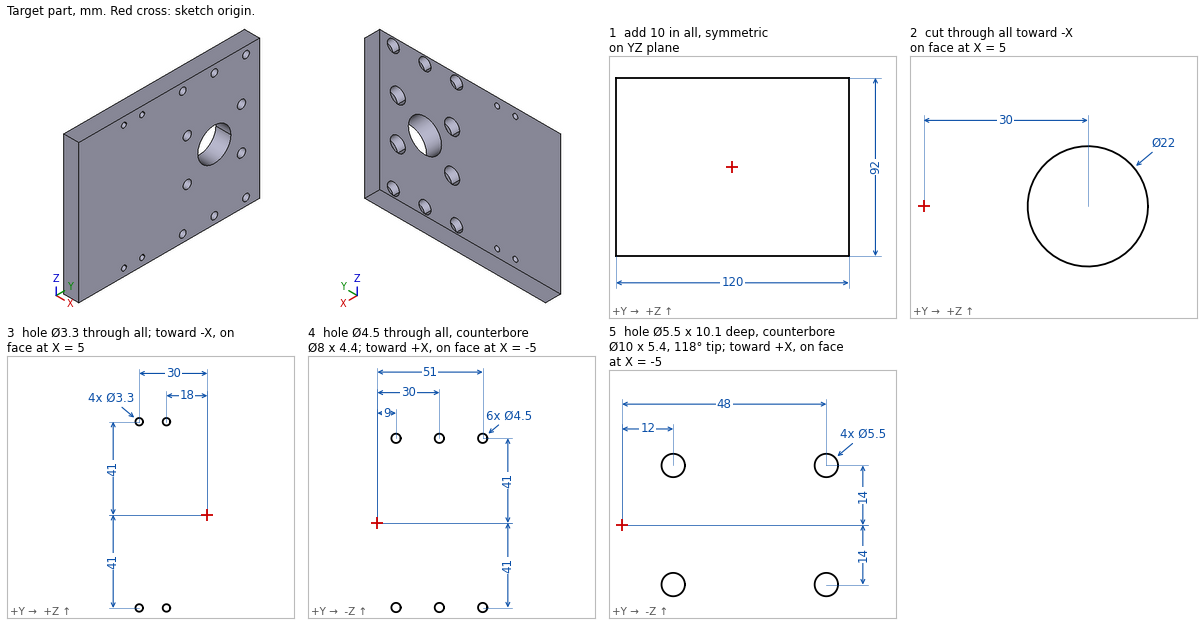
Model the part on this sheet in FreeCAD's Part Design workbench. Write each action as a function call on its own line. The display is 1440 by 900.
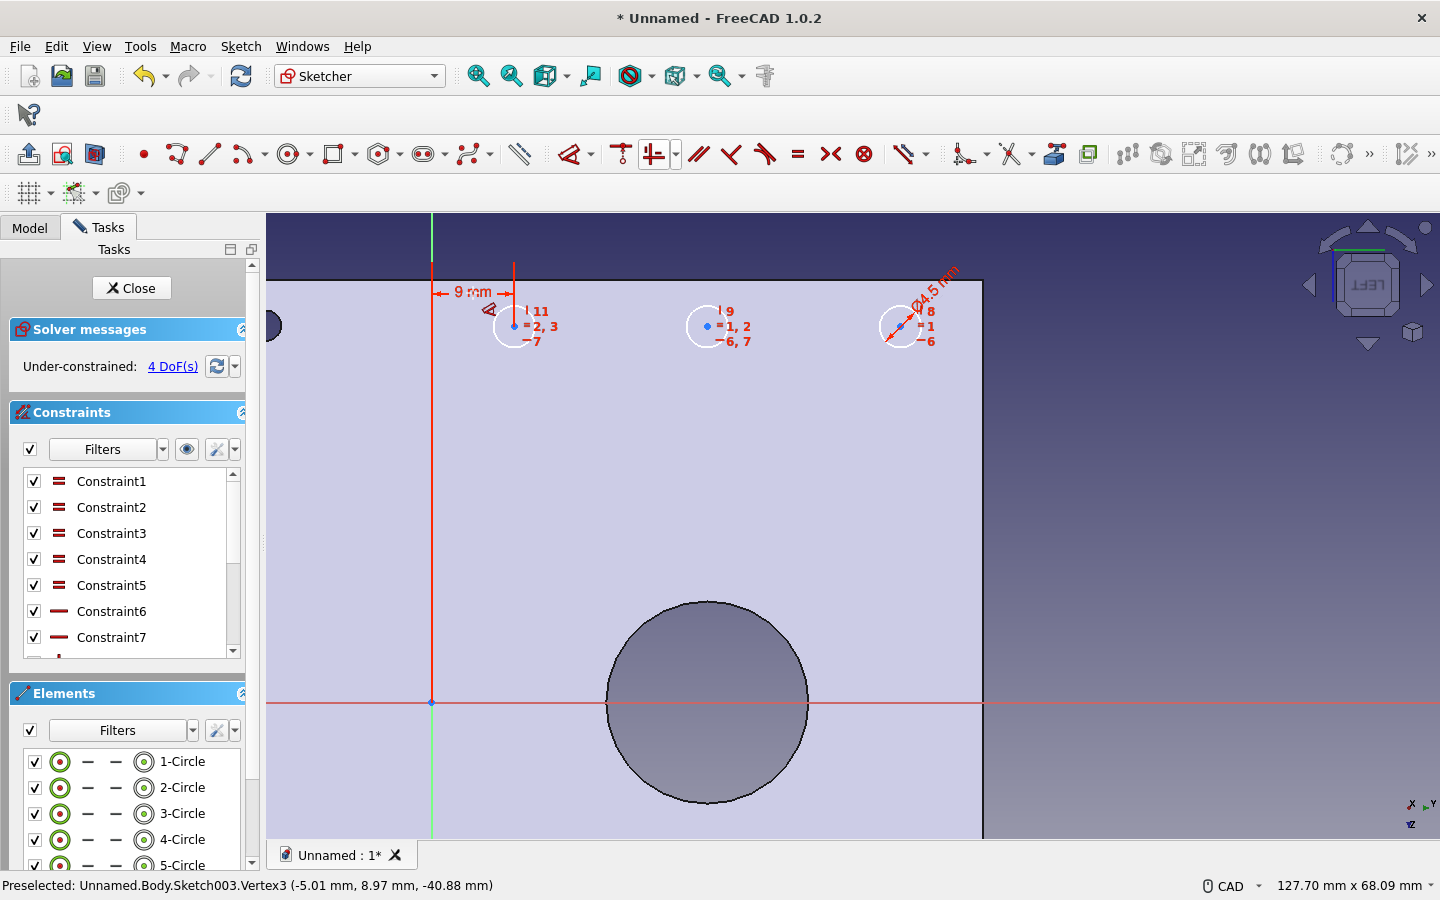
click(900, 327)
click(666, 293)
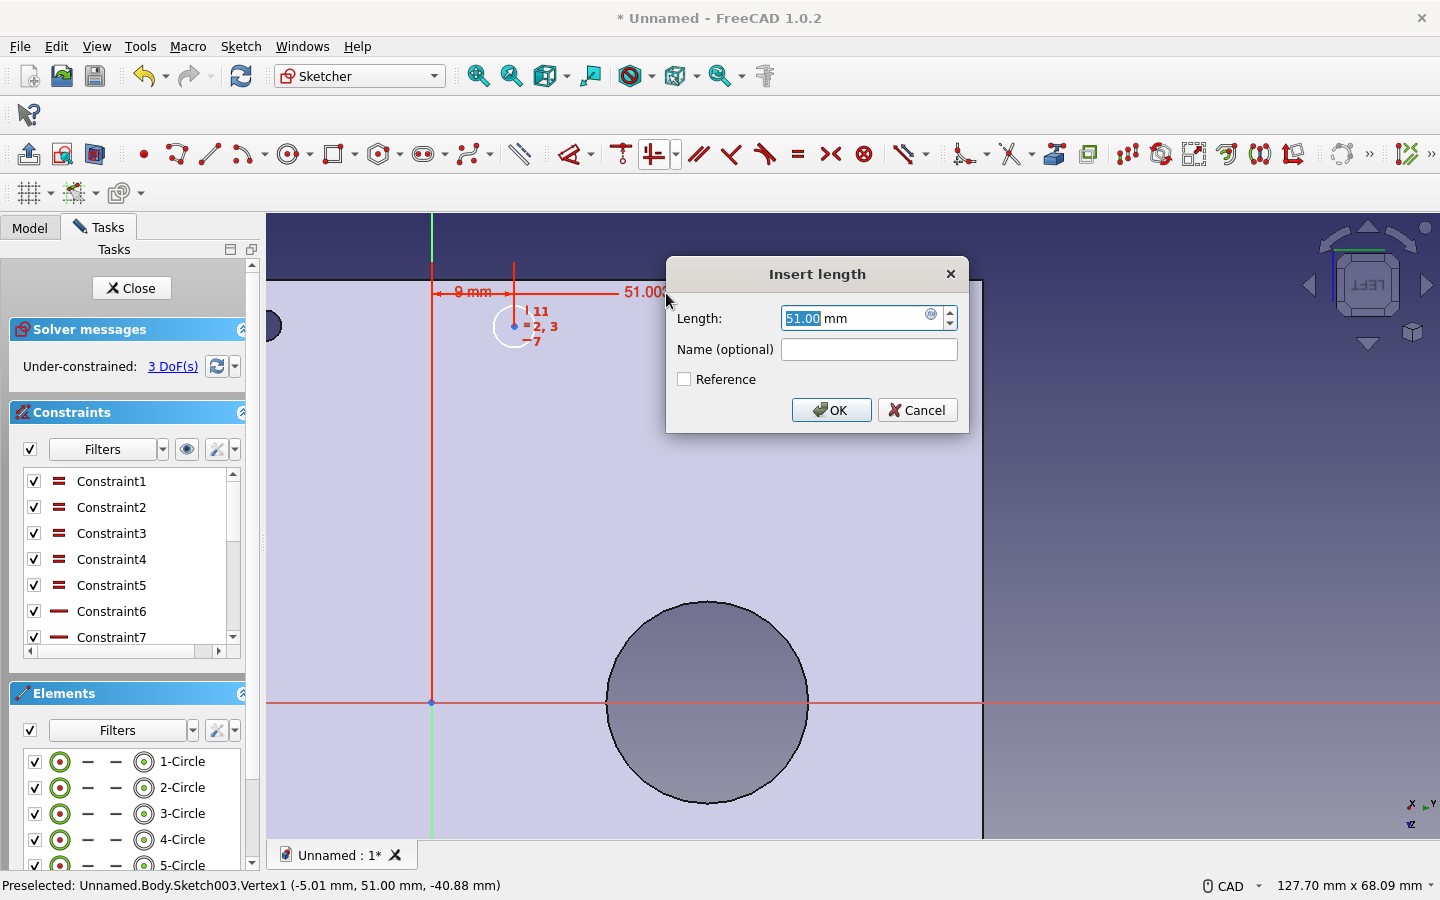
text(51)
key(Return)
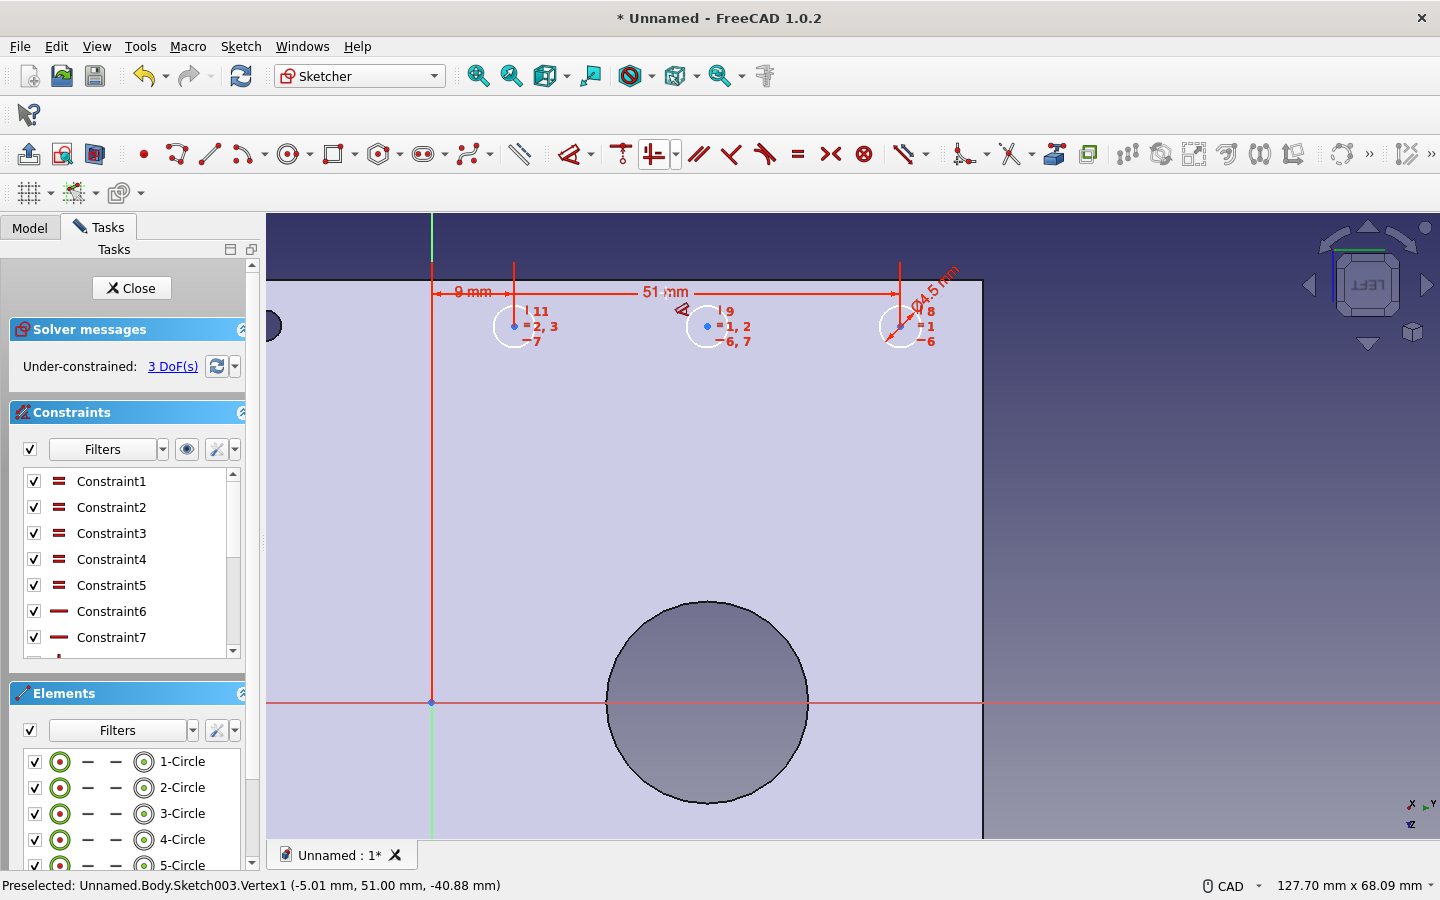
click(900, 327)
click(398, 515)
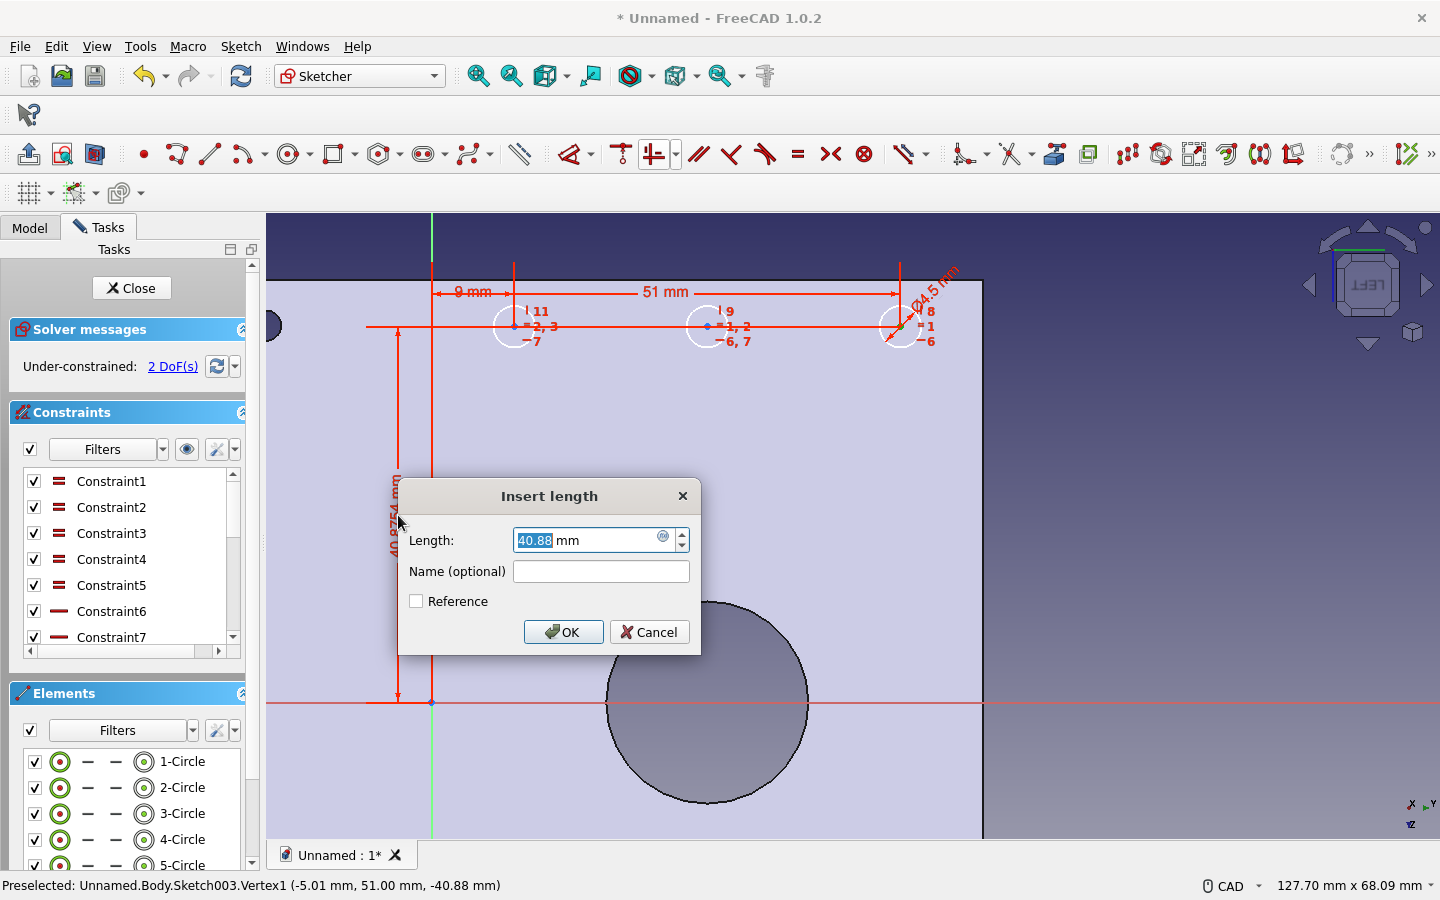
text(41)
key(Return)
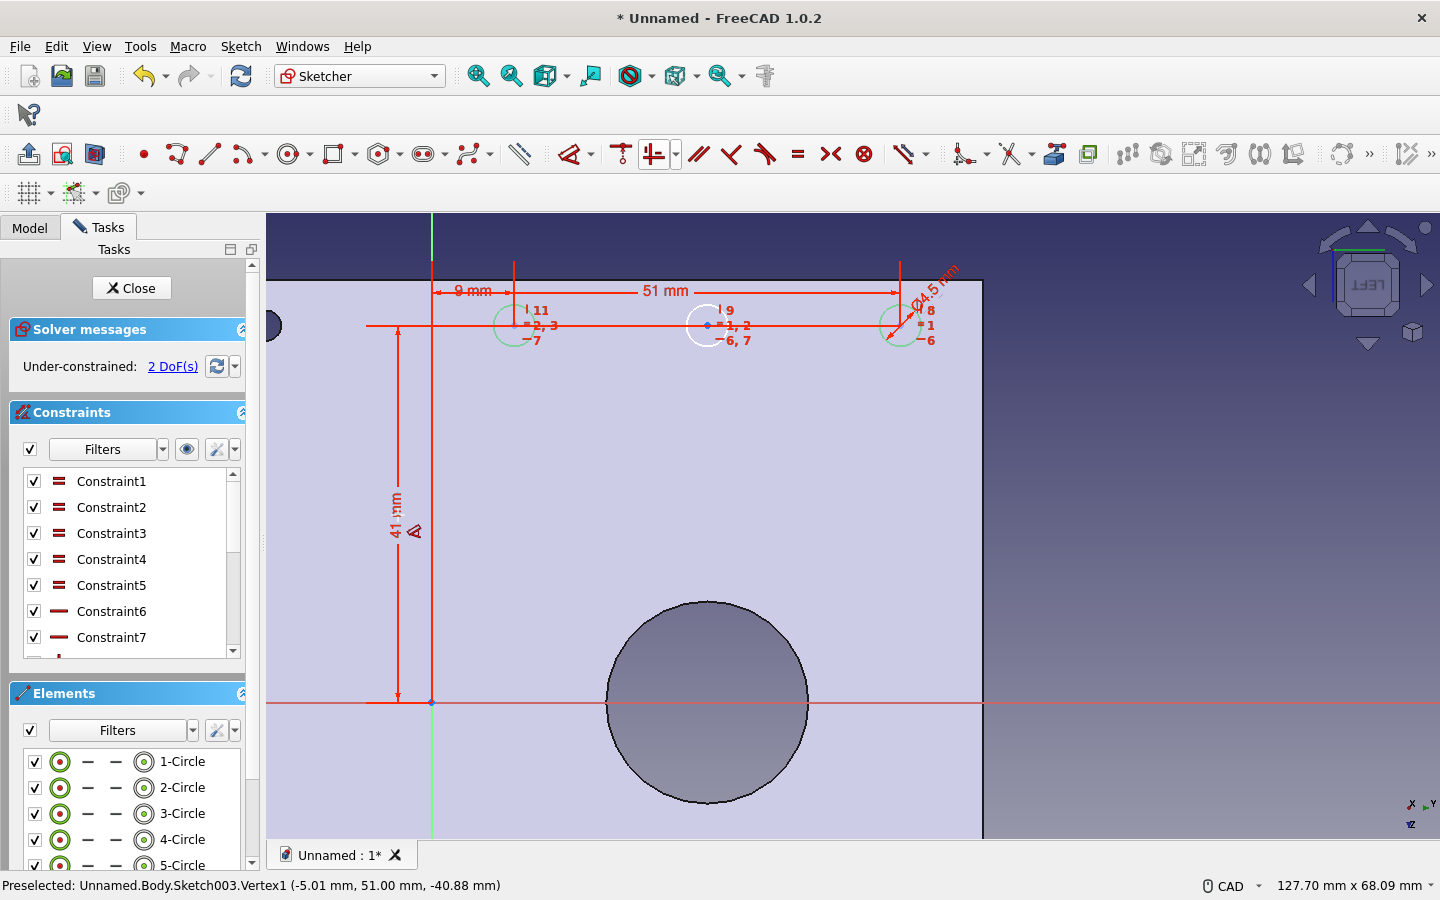
click(707, 326)
click(569, 292)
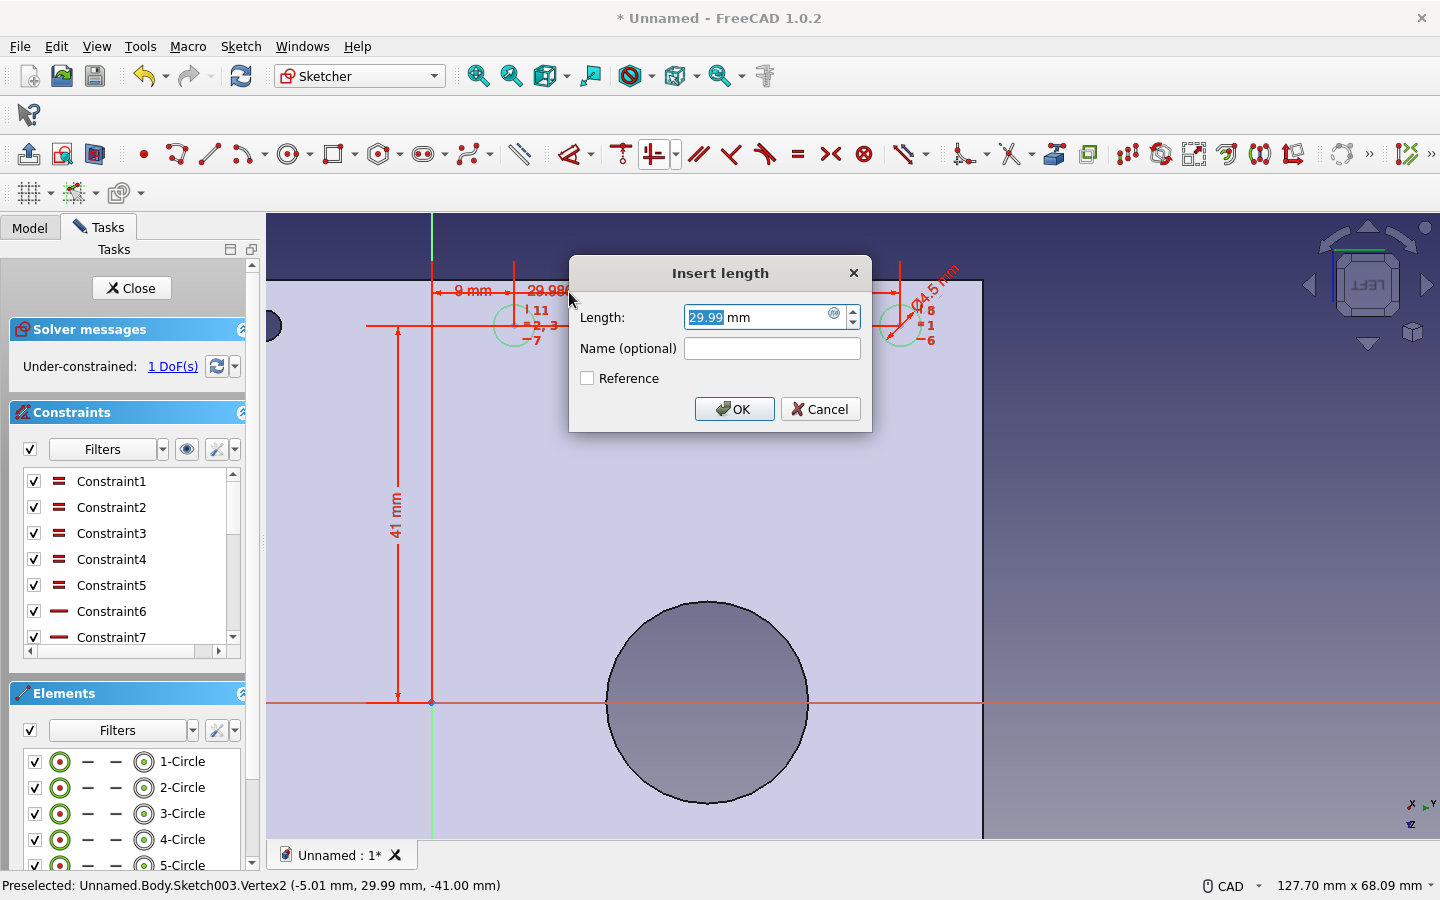
text(30)
key(Return)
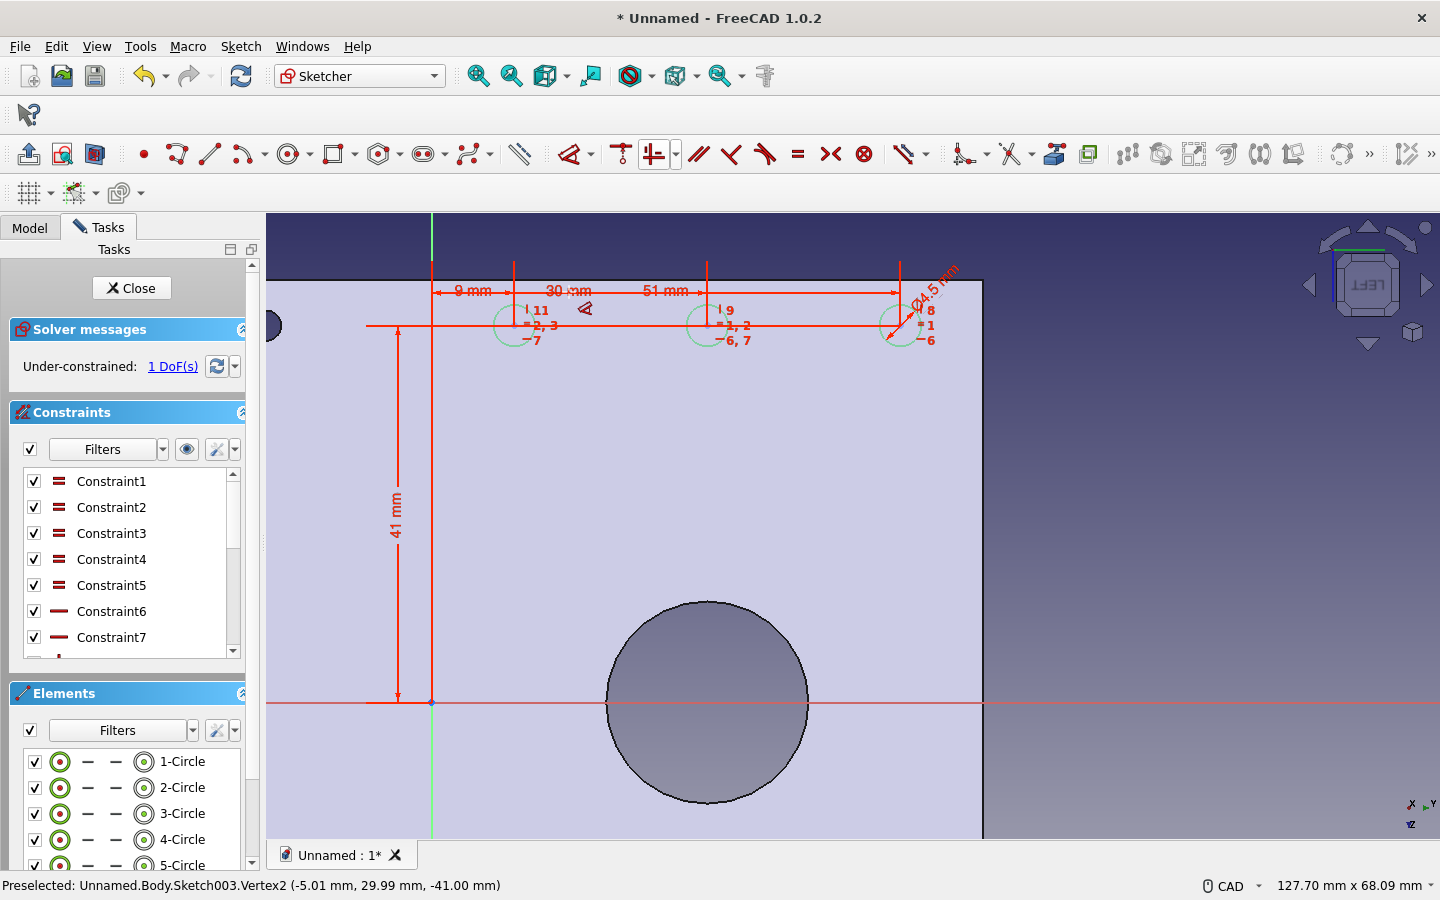
scroll(916, 311, down, 3)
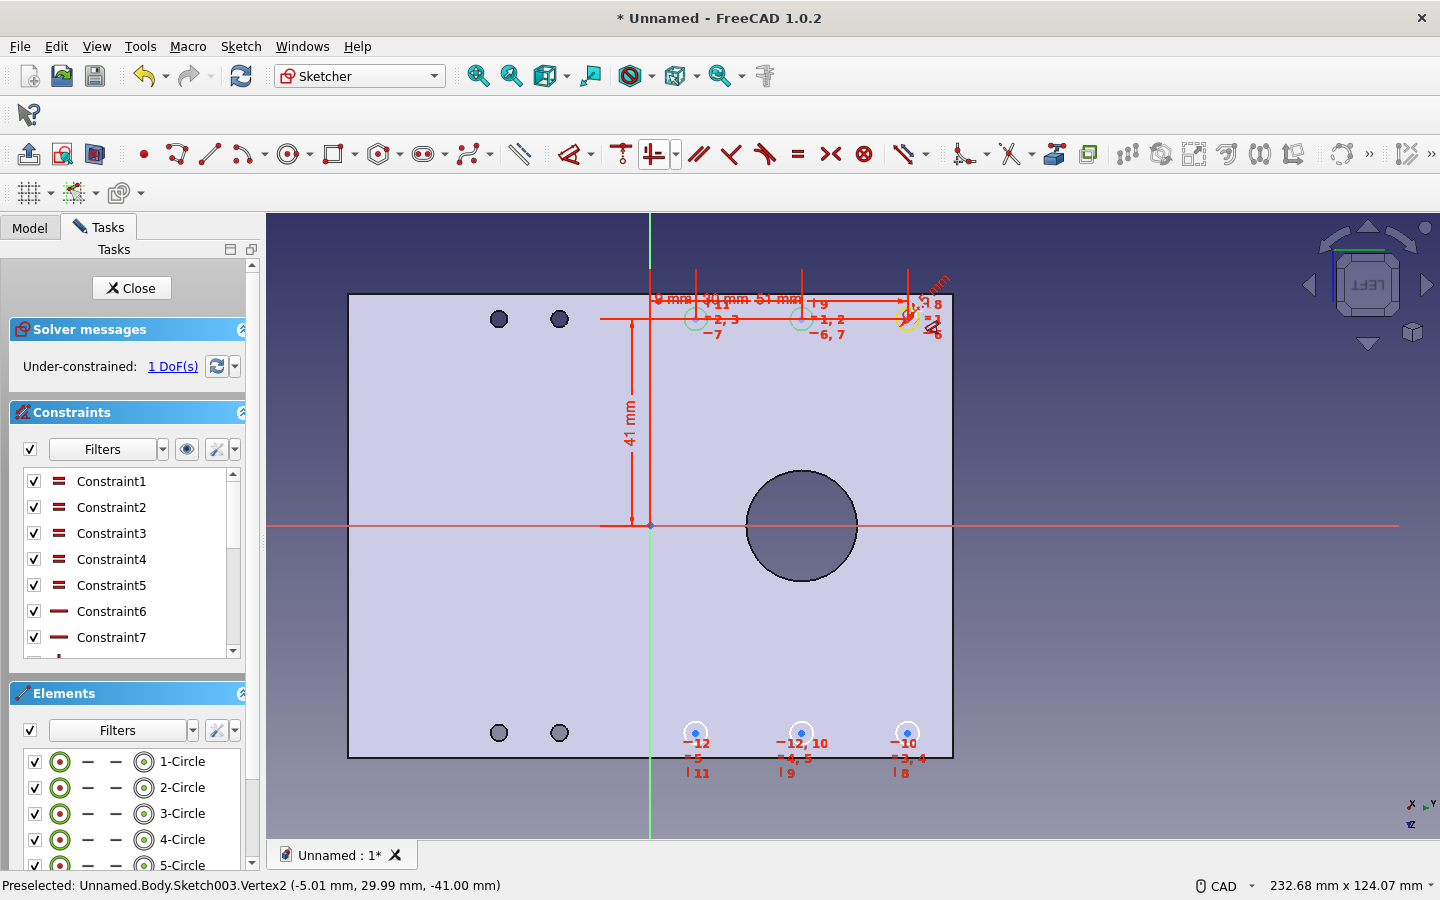
click(908, 733)
click(616, 630)